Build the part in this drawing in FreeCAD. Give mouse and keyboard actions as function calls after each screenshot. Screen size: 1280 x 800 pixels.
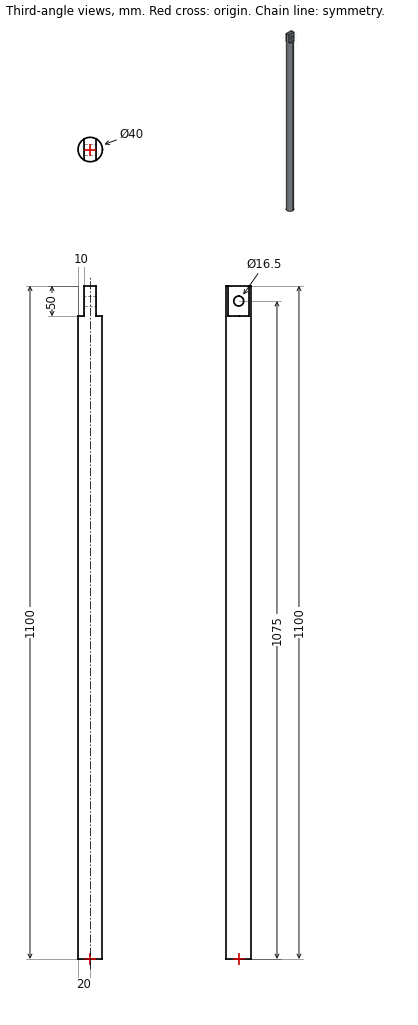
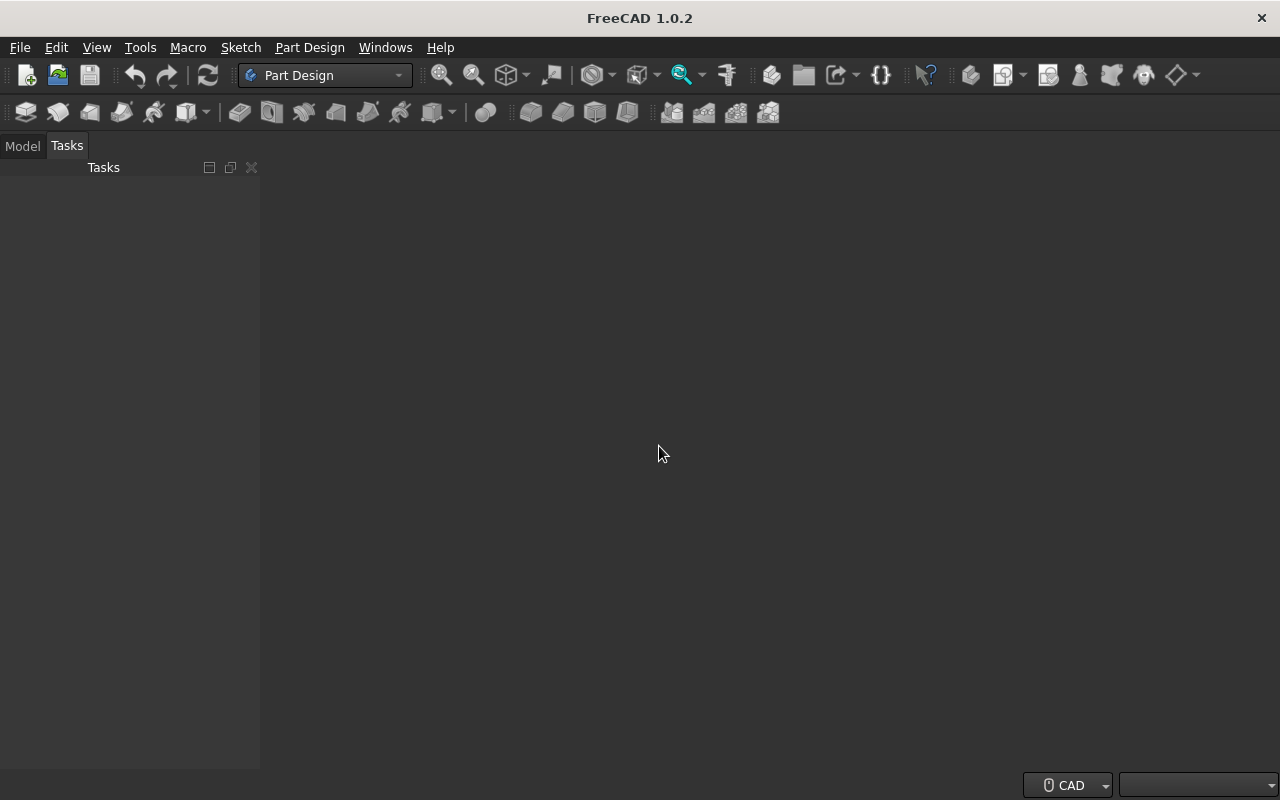
click(26, 76)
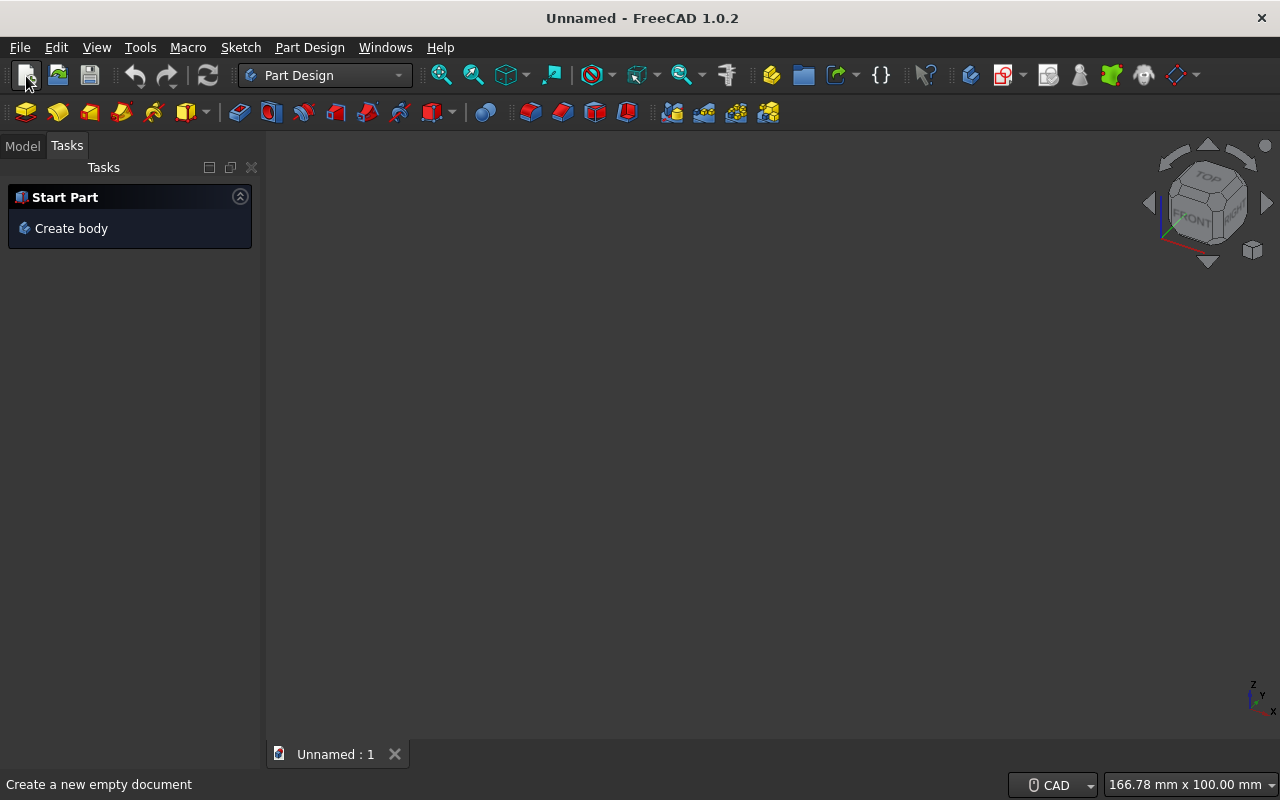
click(1004, 76)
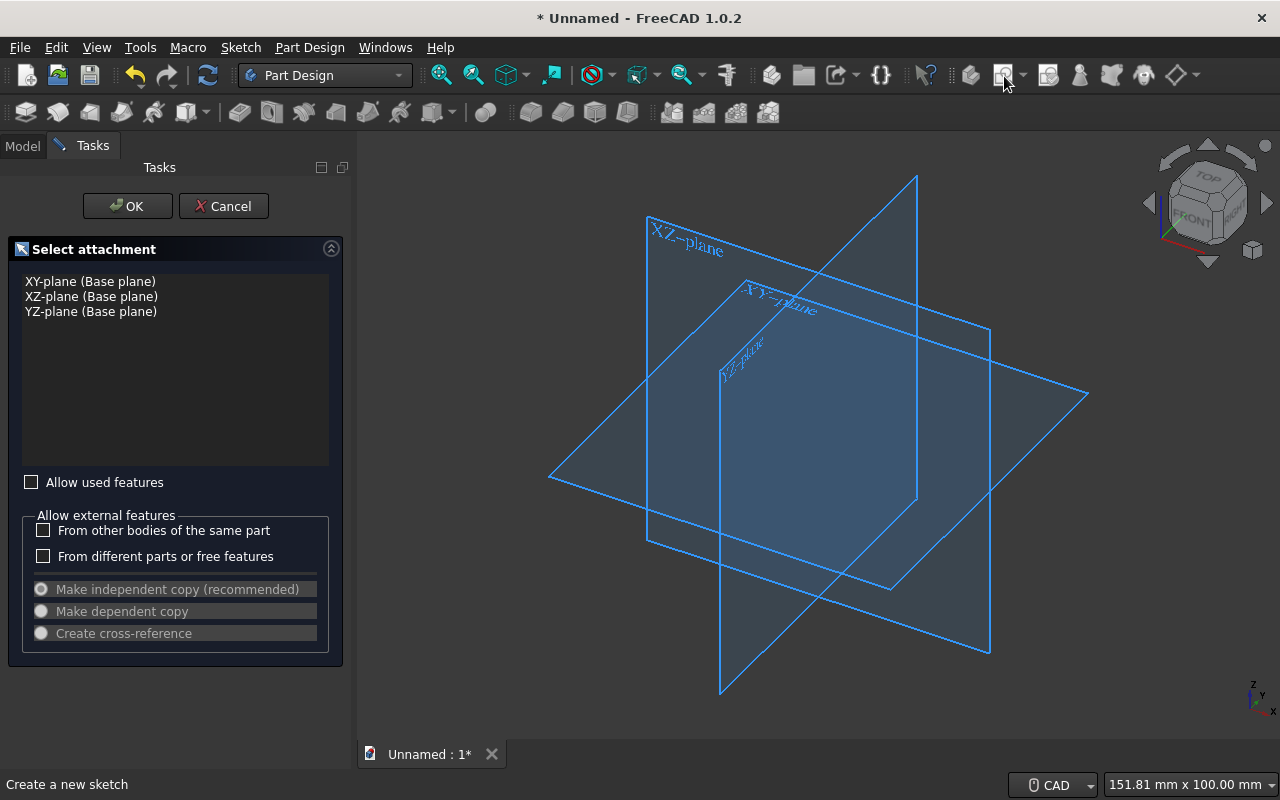
click(82, 282)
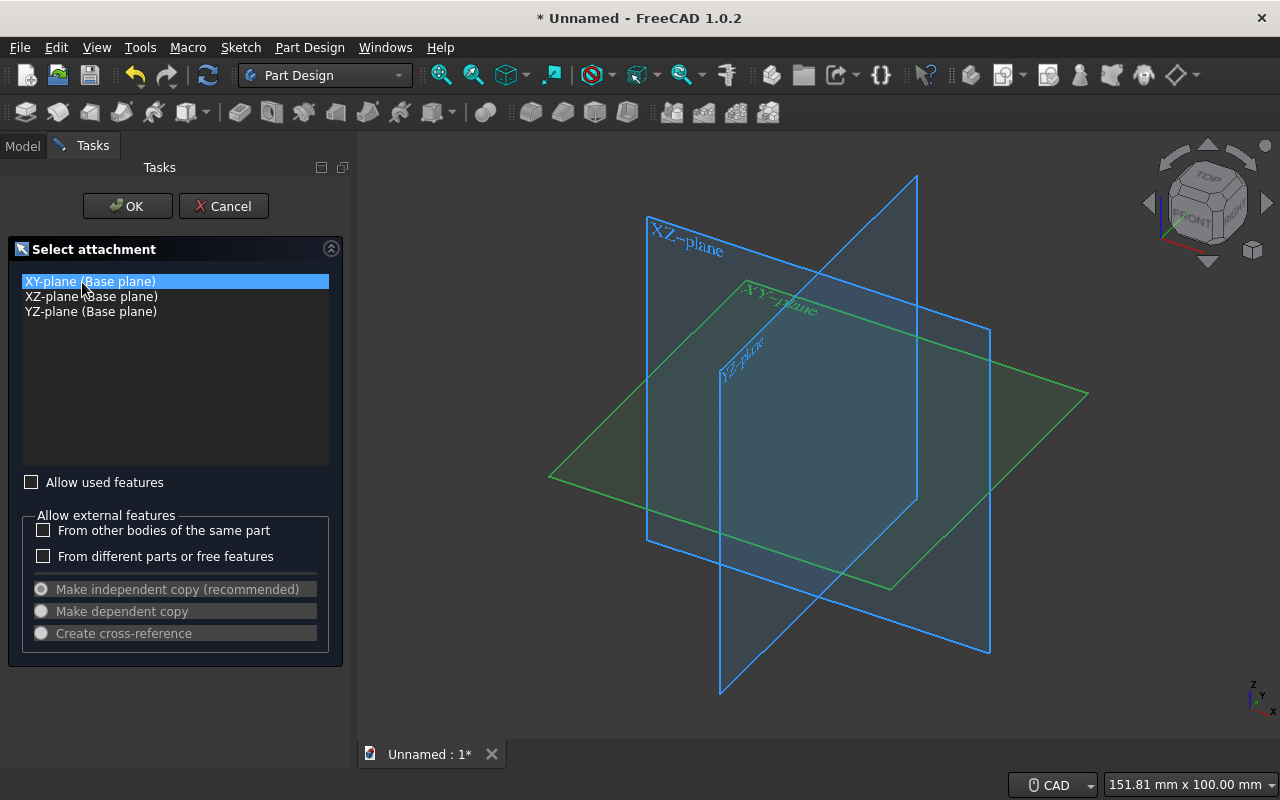
click(128, 206)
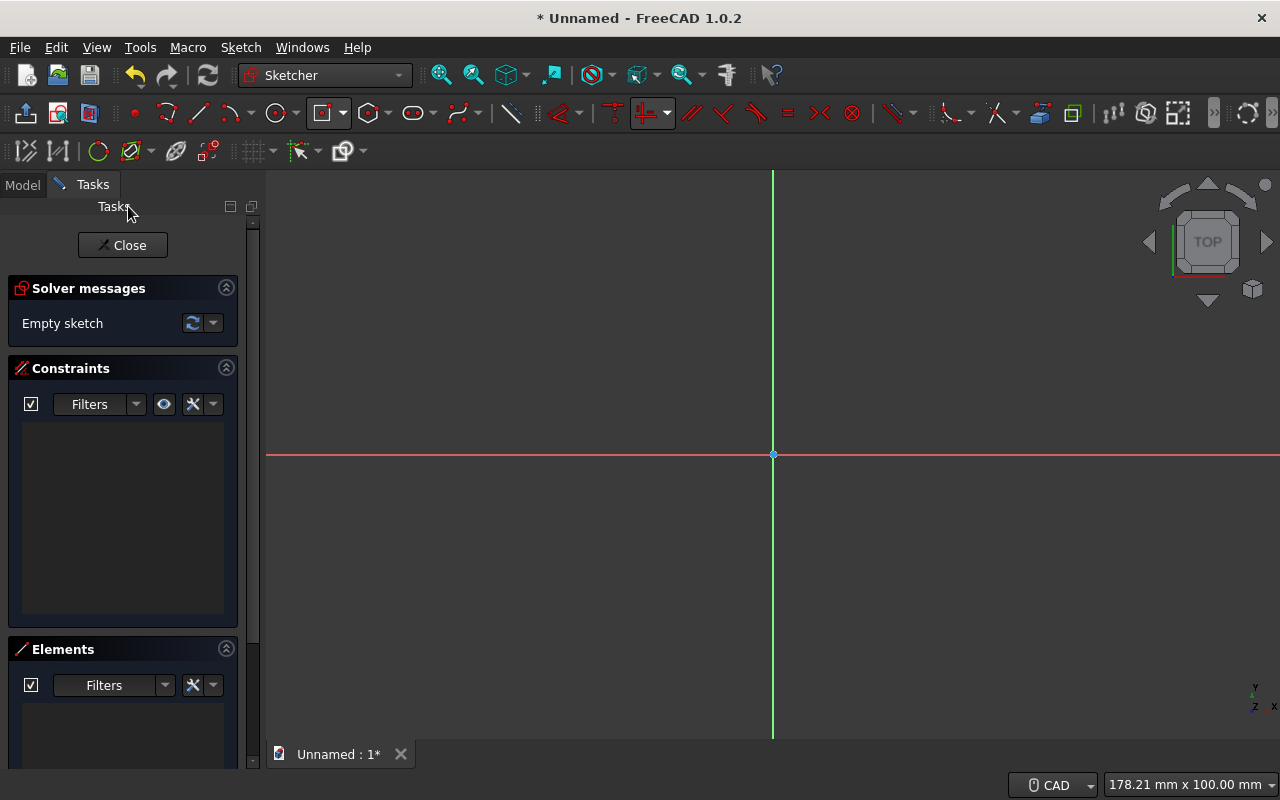
scroll(912, 455, up, 2)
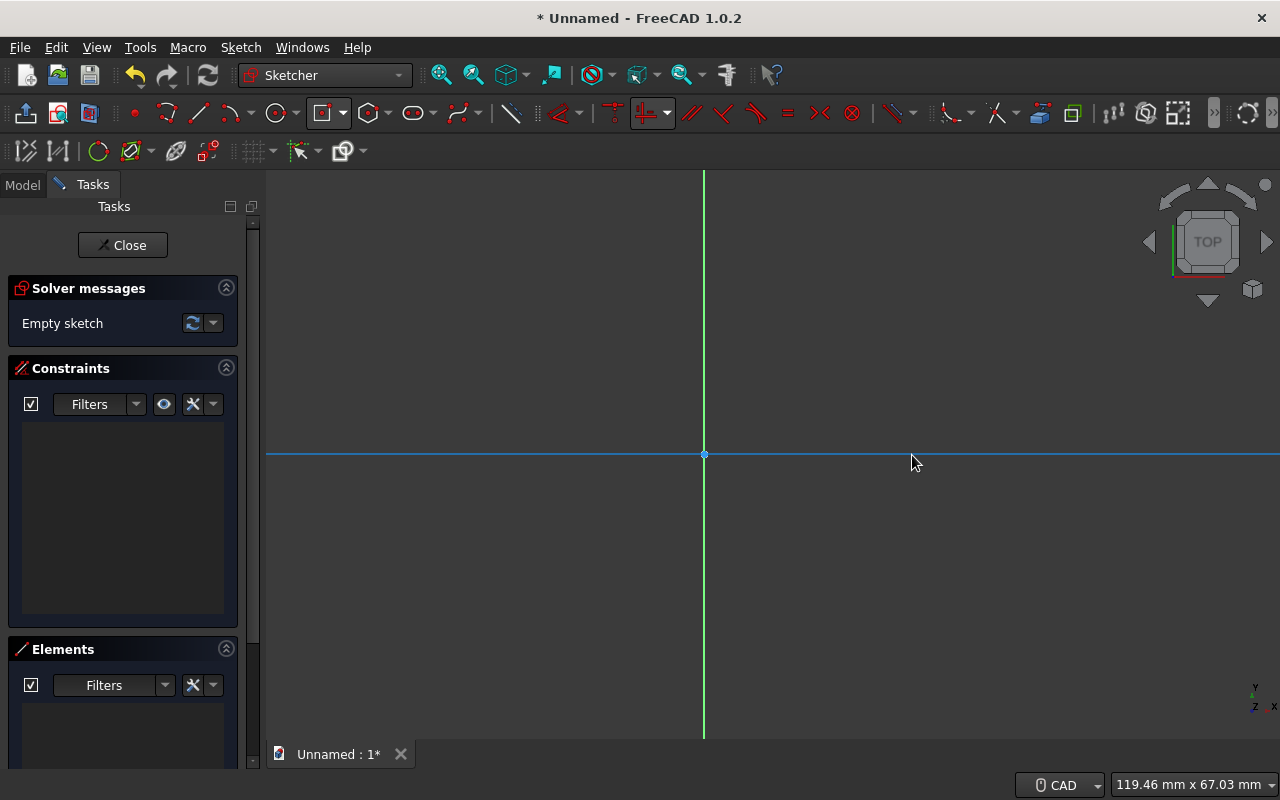
click(276, 114)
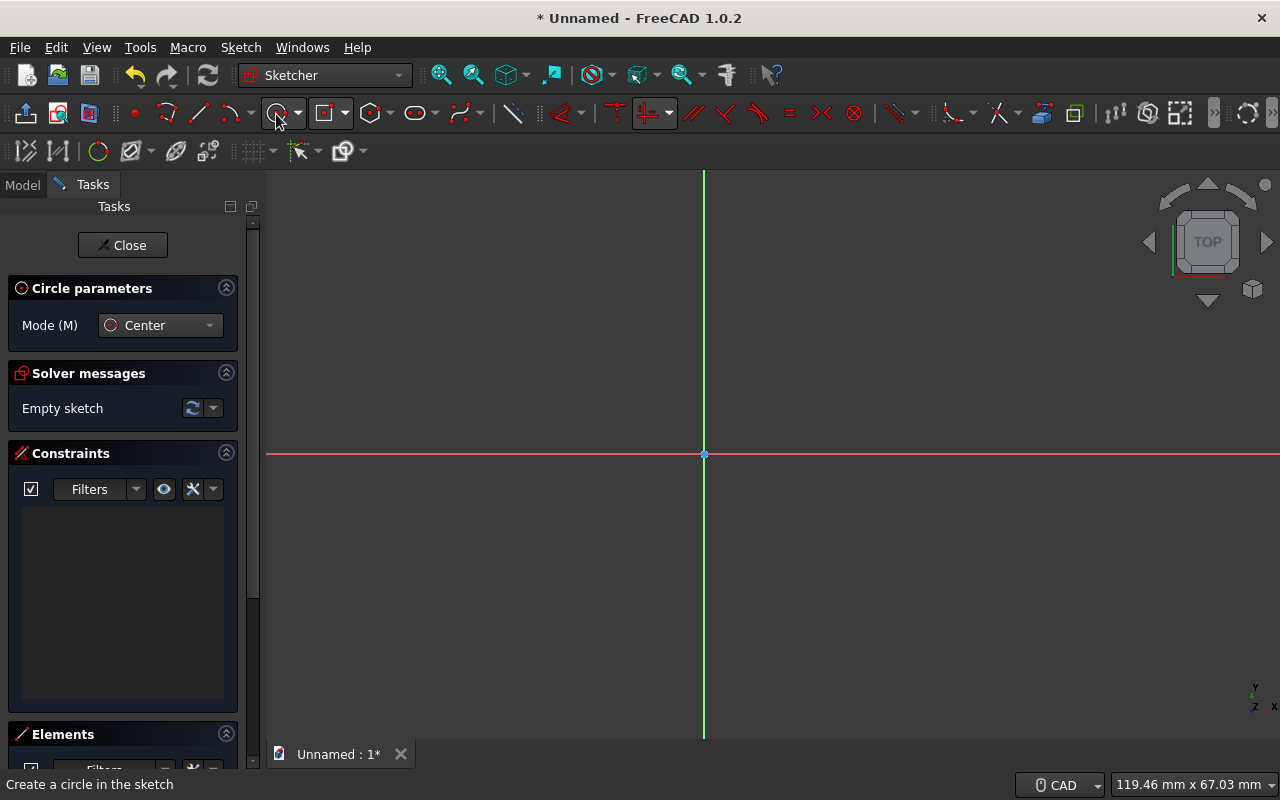
click(704, 454)
click(824, 334)
key(Escape)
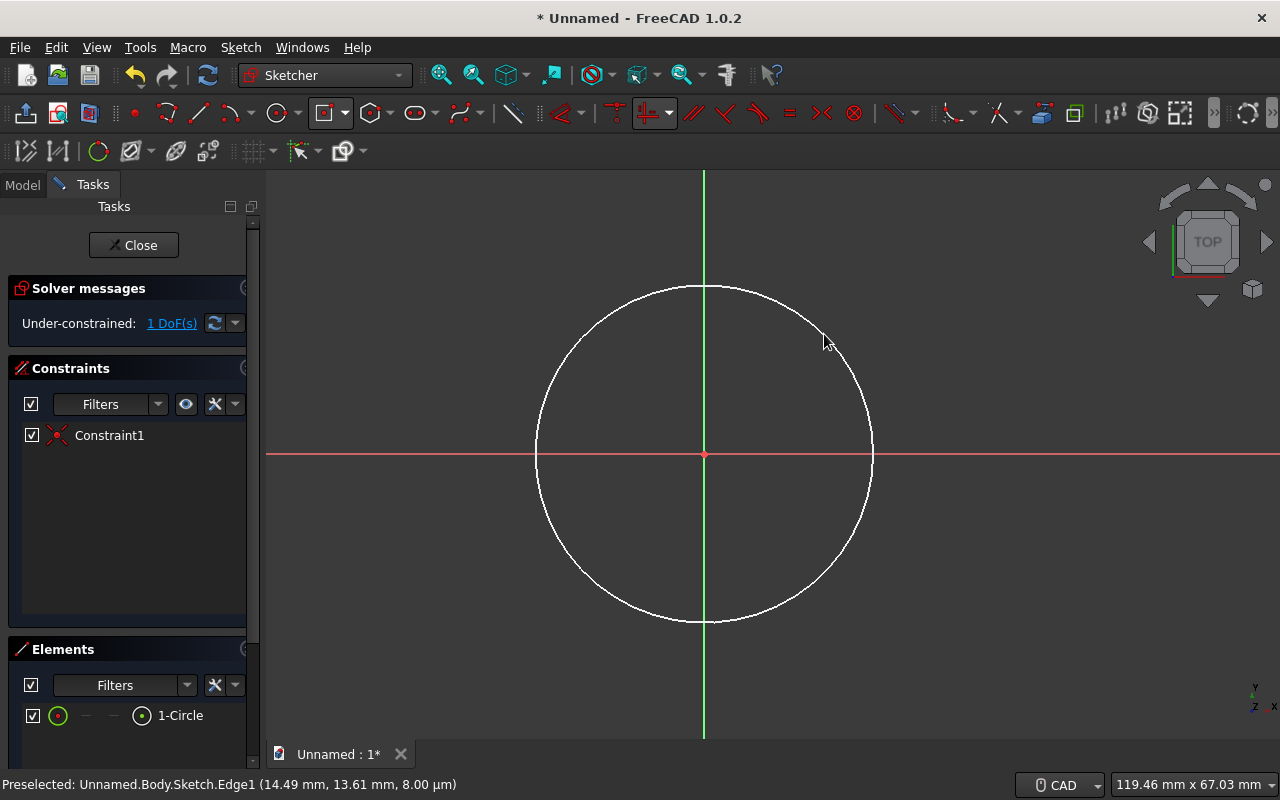
click(560, 114)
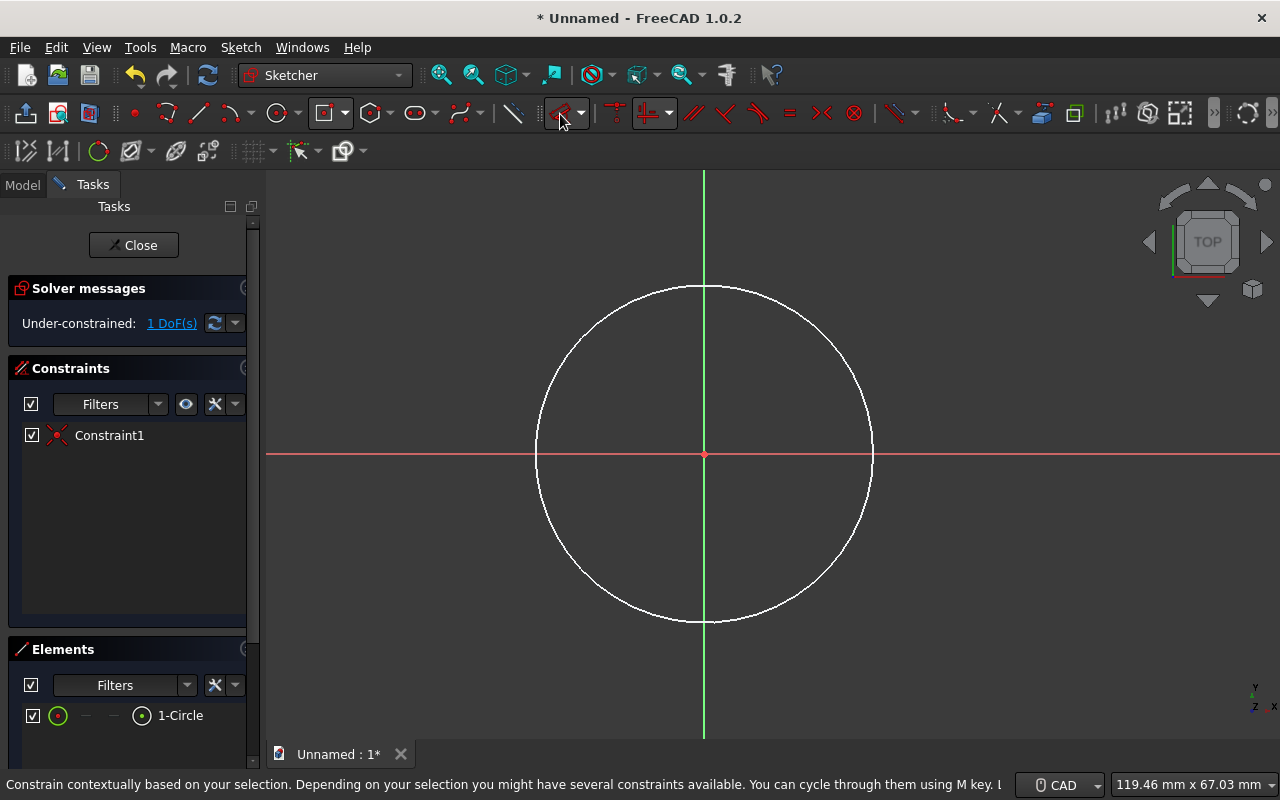
click(823, 334)
click(846, 311)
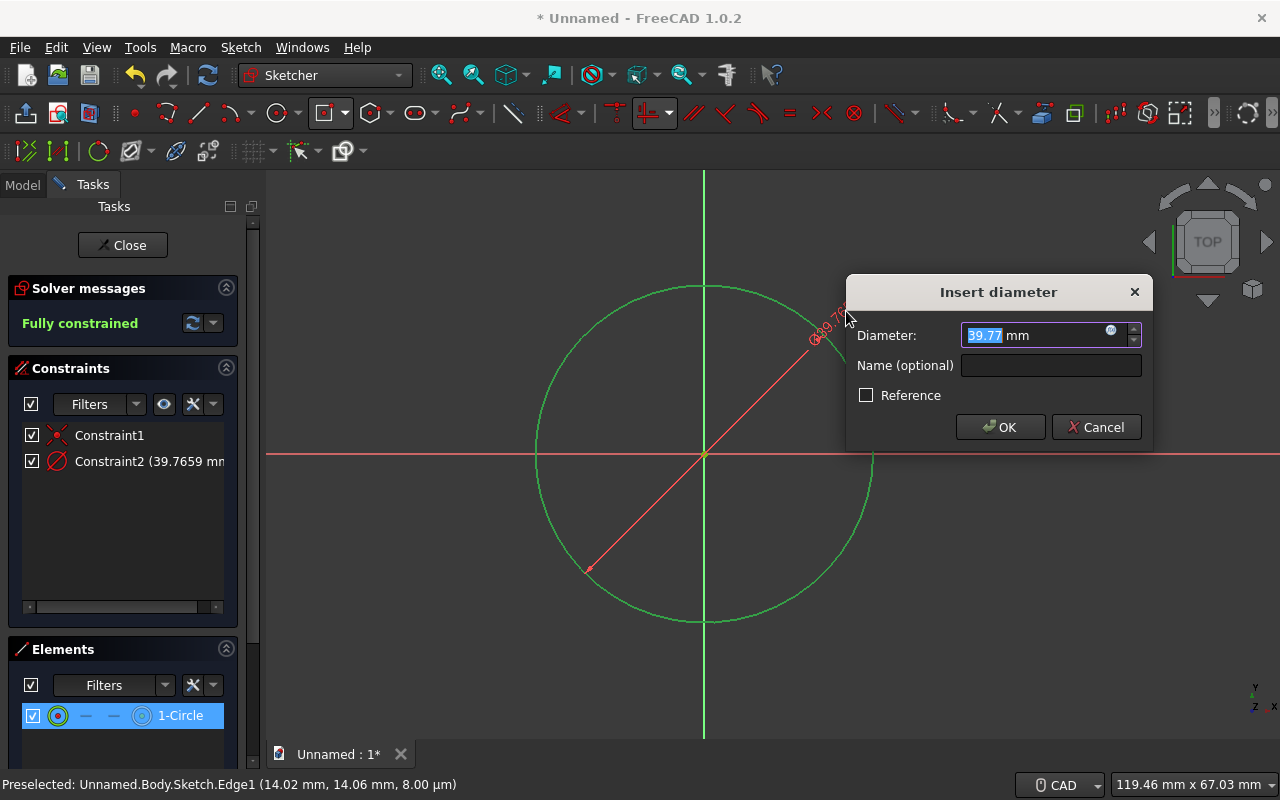
text(40)
key(Return)
key(Escape)